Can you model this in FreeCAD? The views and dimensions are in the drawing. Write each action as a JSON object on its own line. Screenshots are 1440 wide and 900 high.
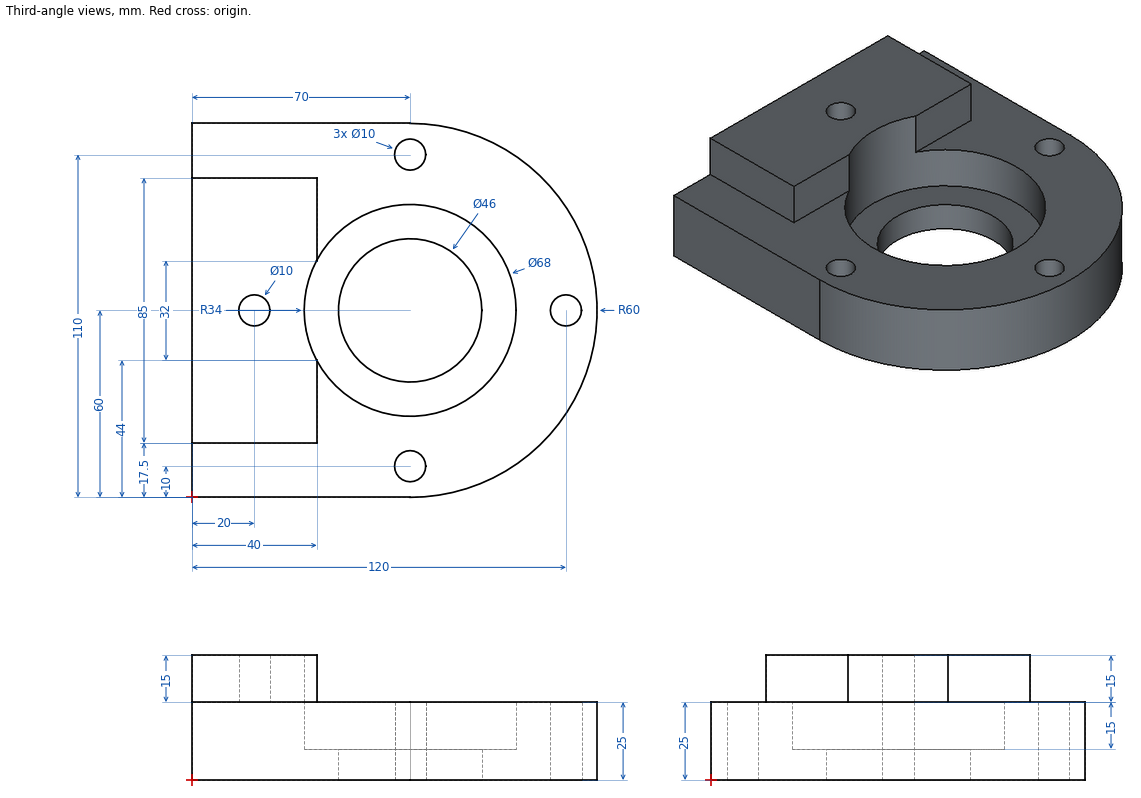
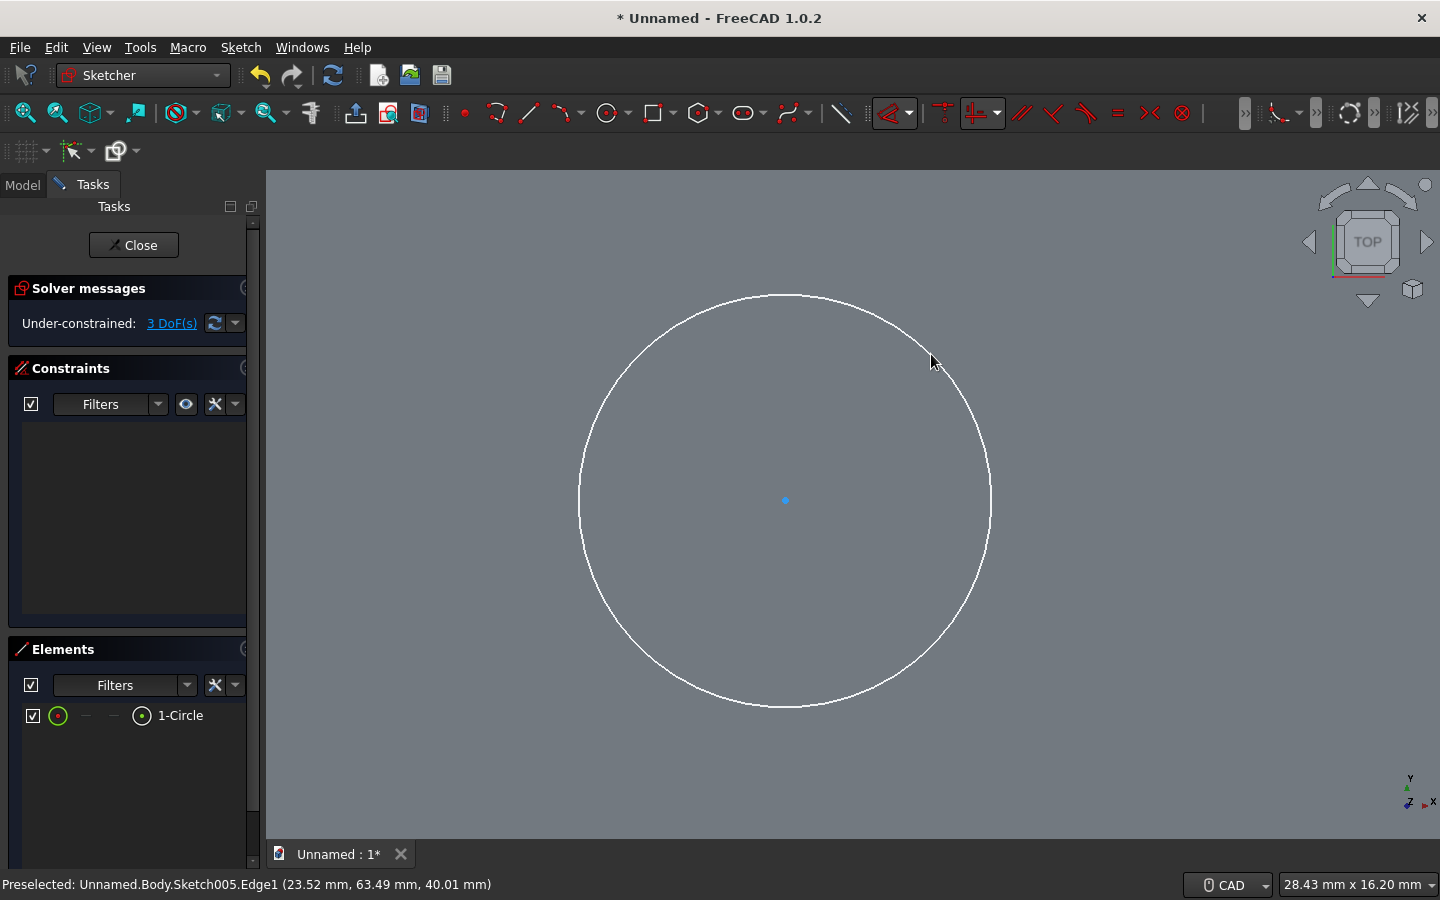
{"action": "left_click", "coordinate": [931, 355]}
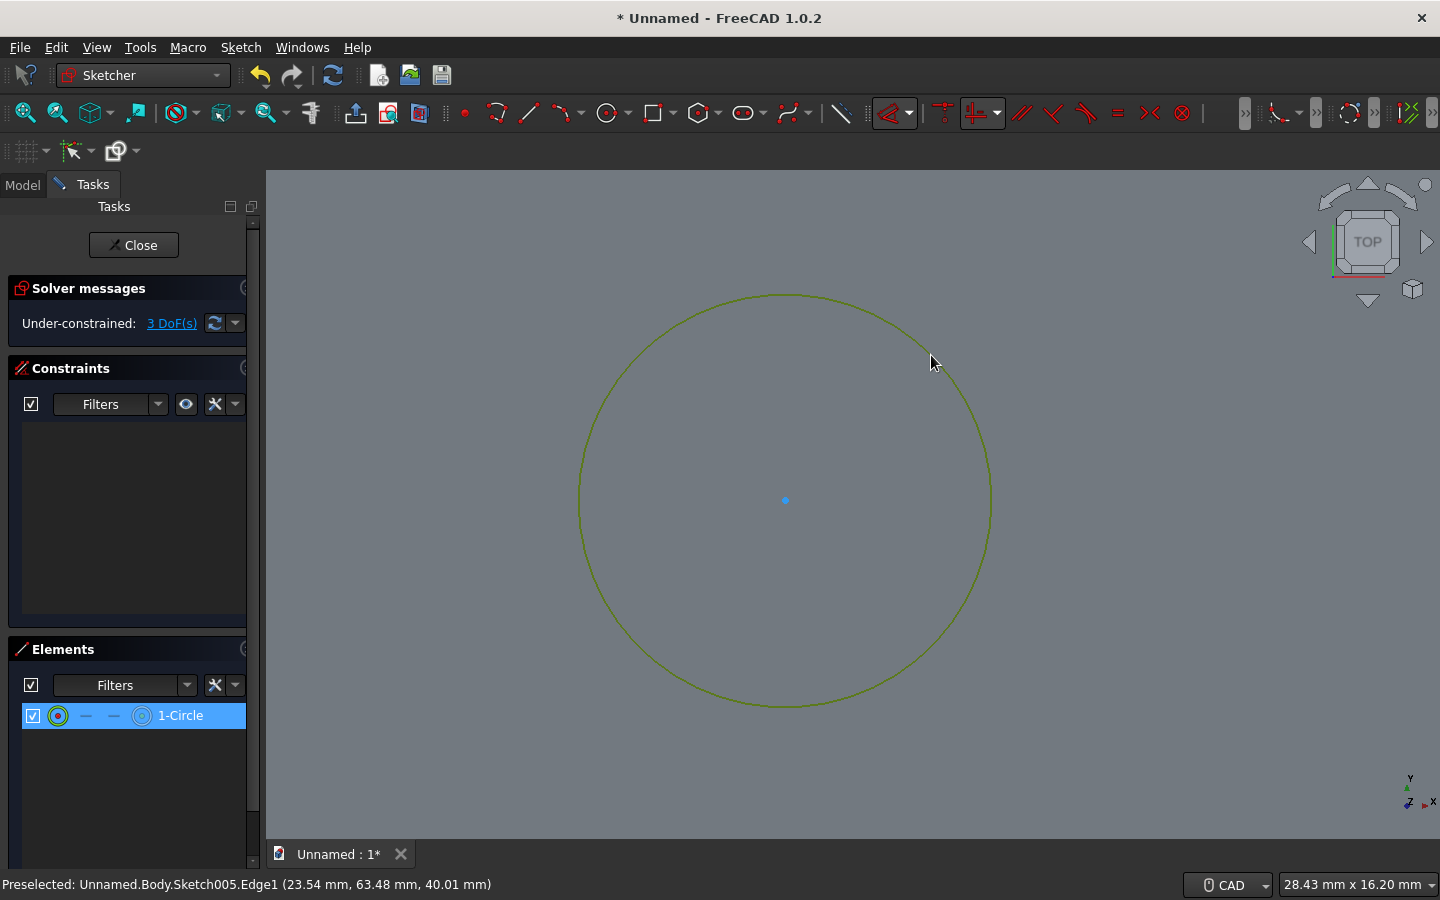
{"action": "key", "text": "k o"}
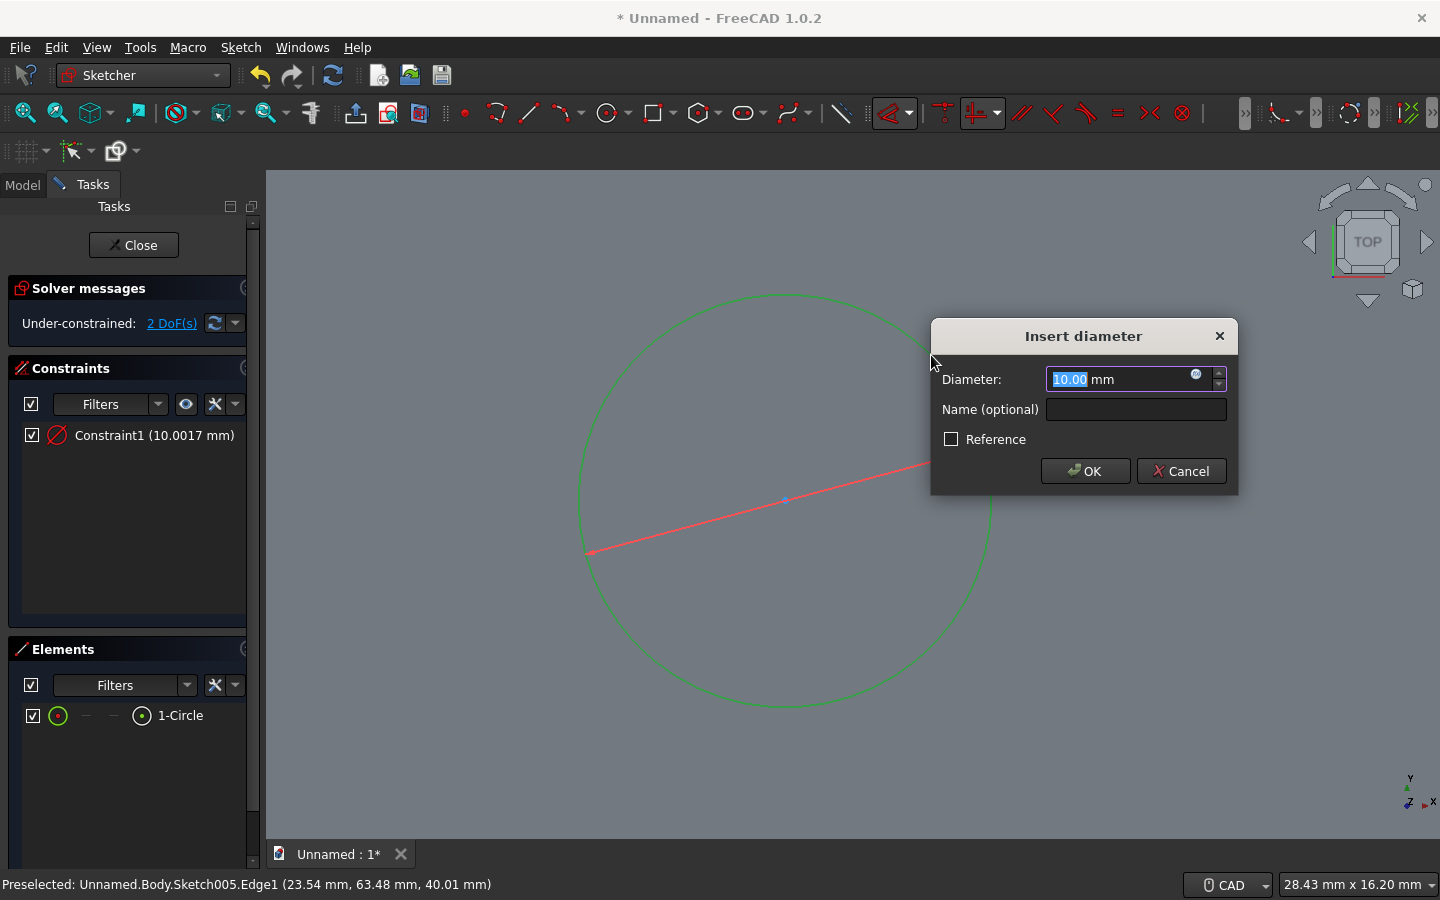
{"action": "type", "text": "10"}
{"action": "key", "text": "Return"}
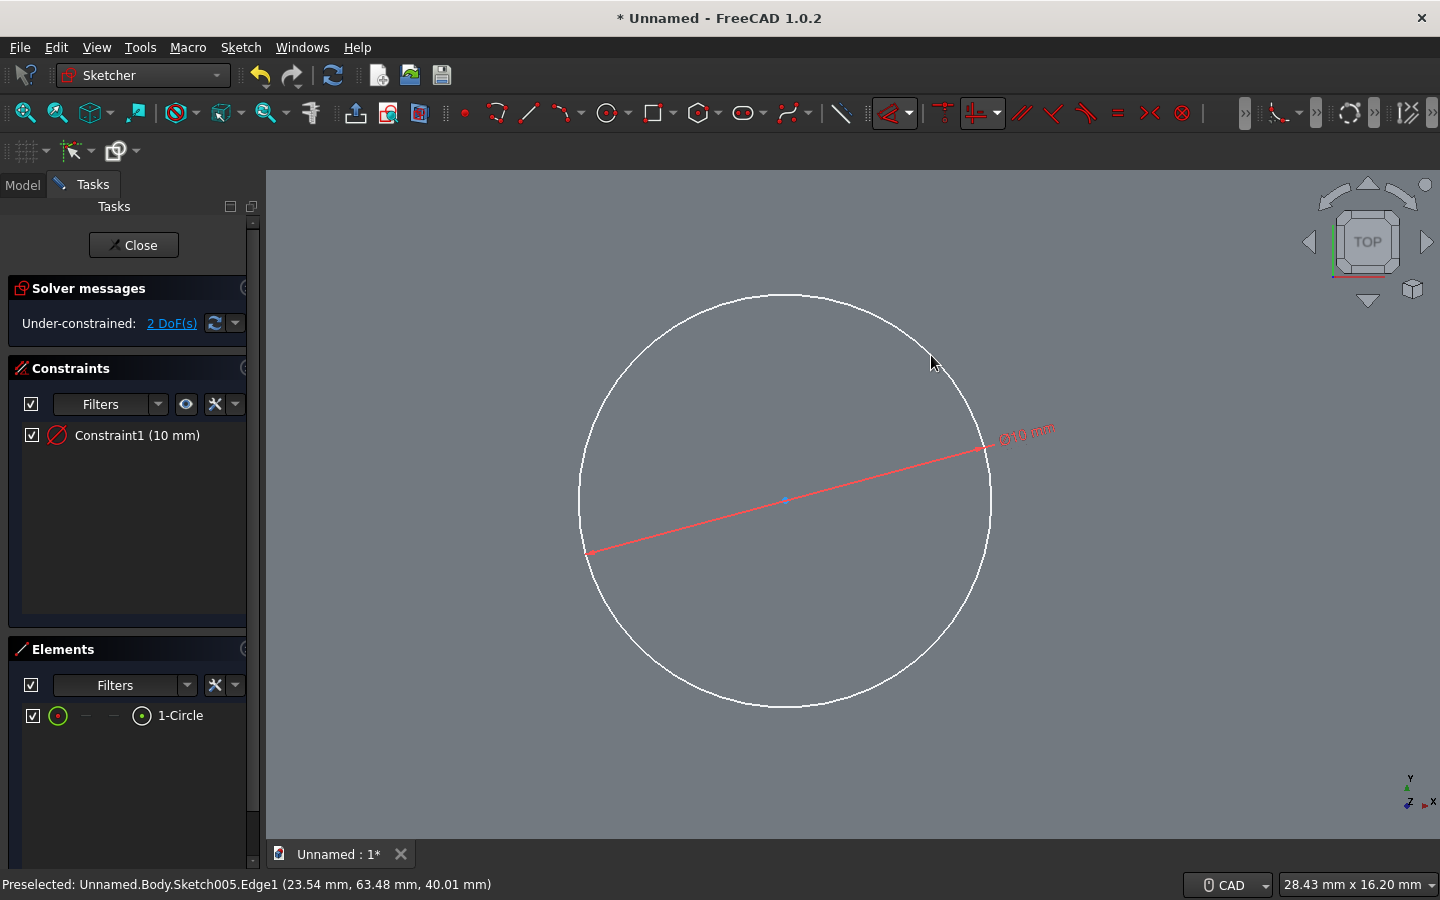
{"action": "left_click", "coordinate": [785, 501]}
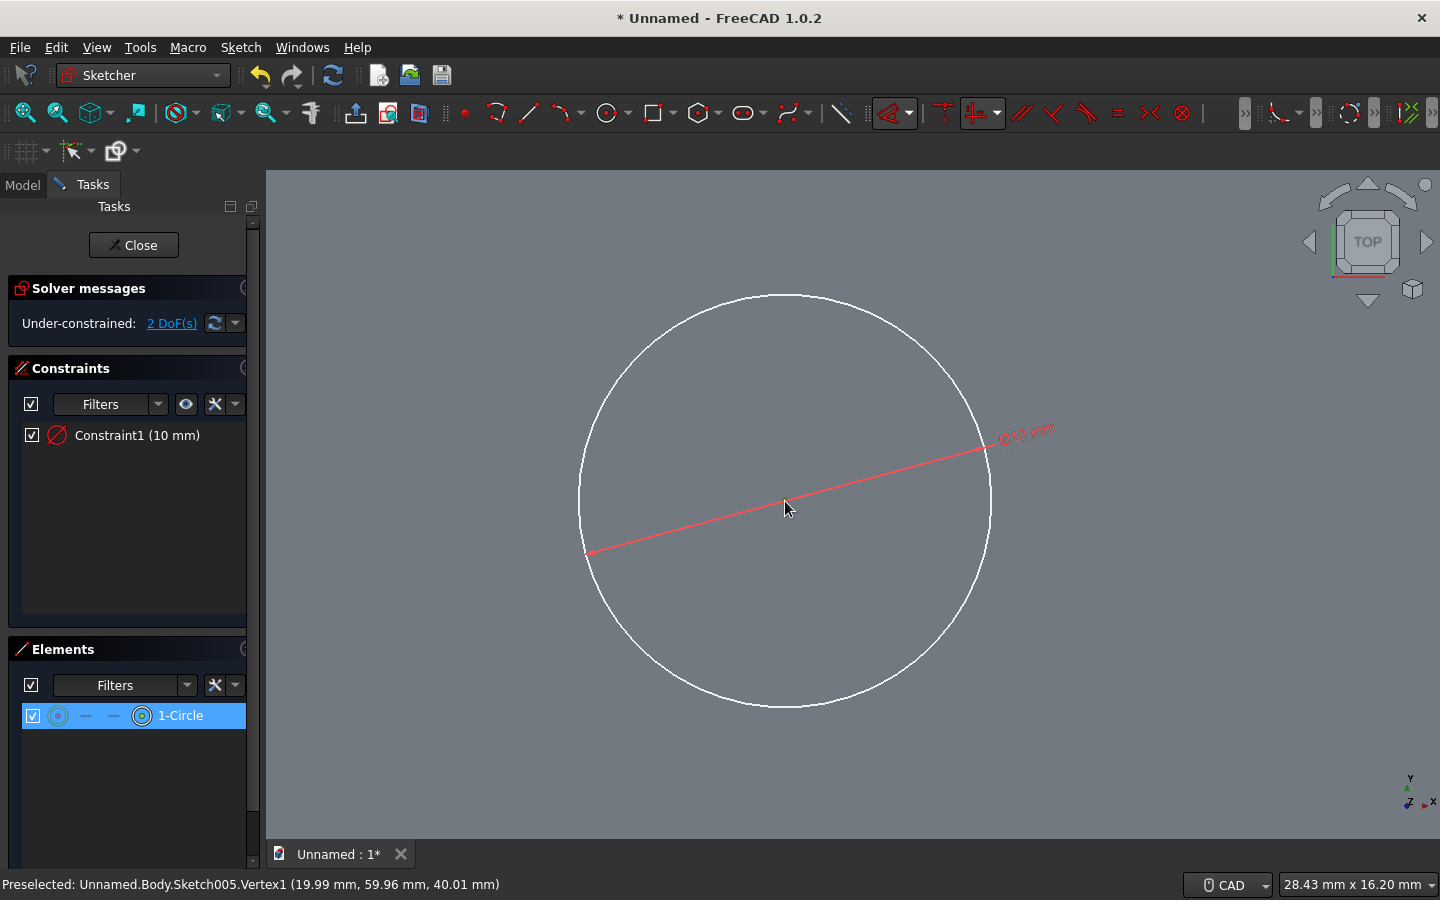
{"action": "left_click", "coordinate": [912, 114]}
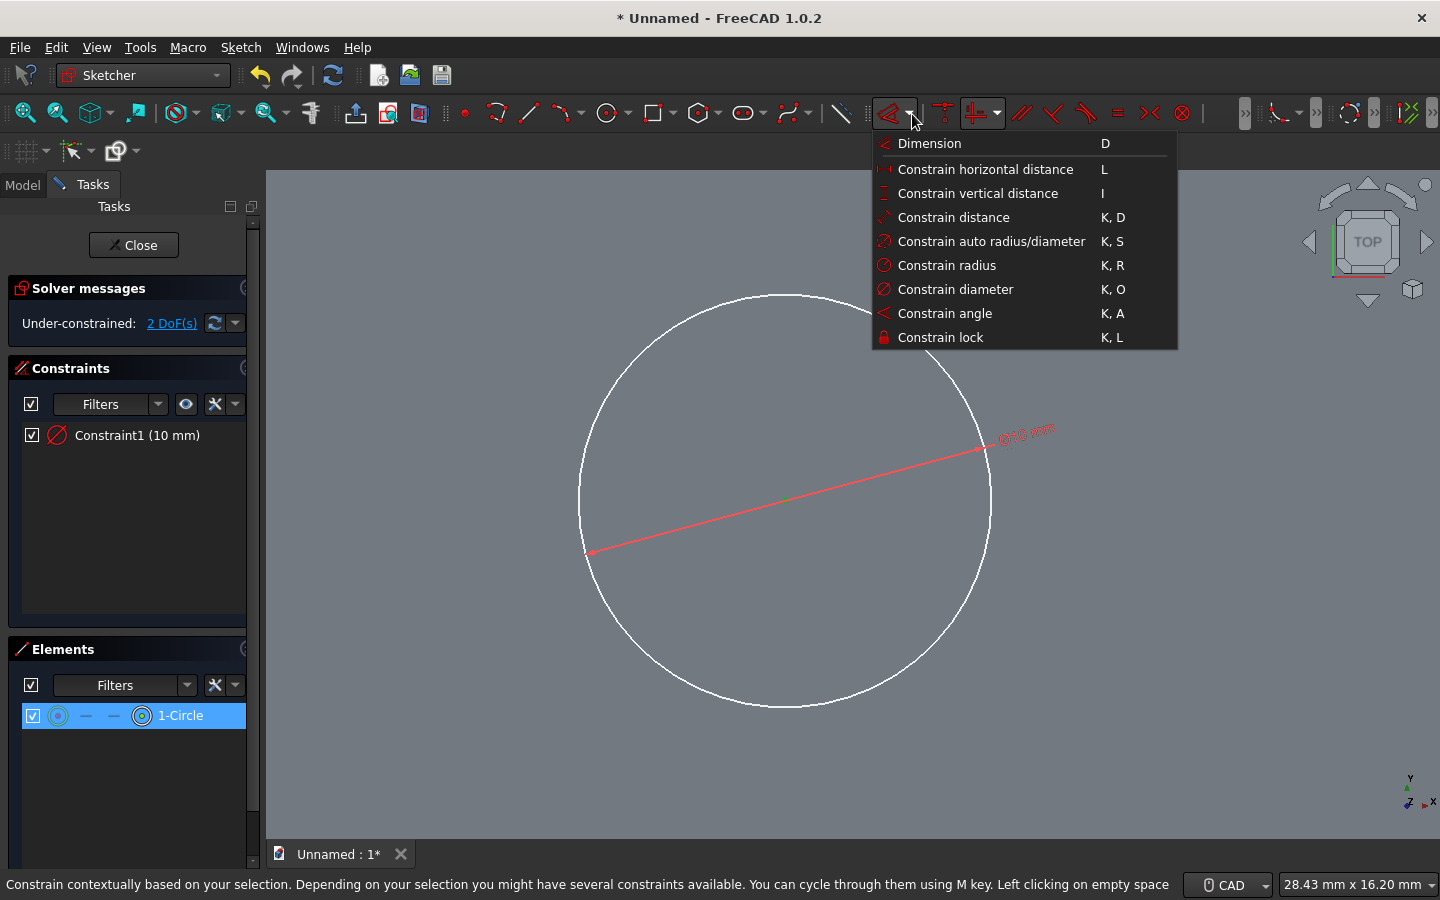
{"action": "left_click", "coordinate": [1025, 169]}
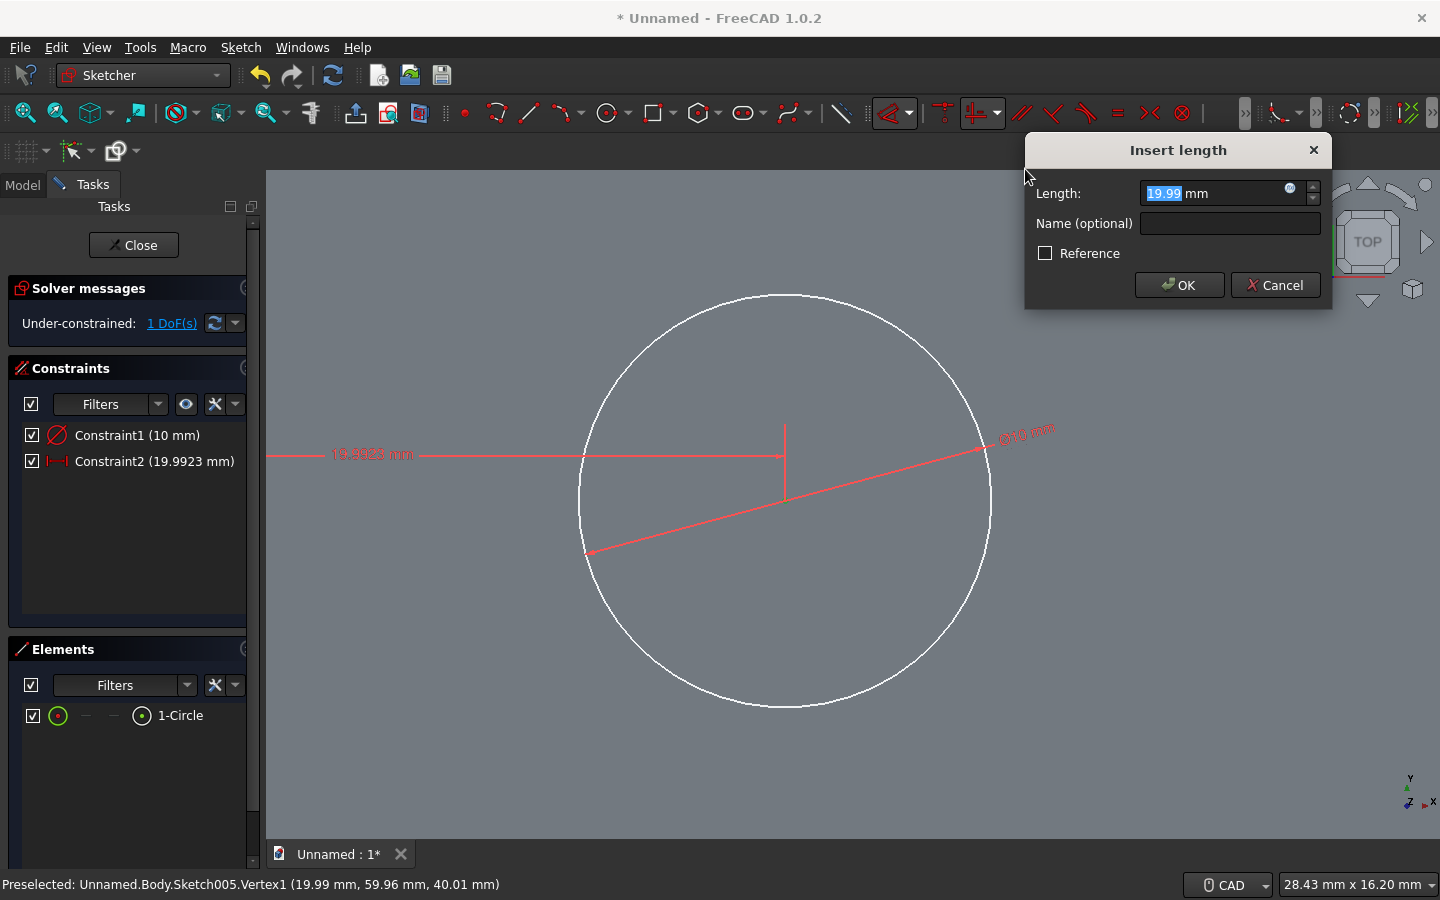
{"action": "type", "text": "20"}
{"action": "key", "text": "Return"}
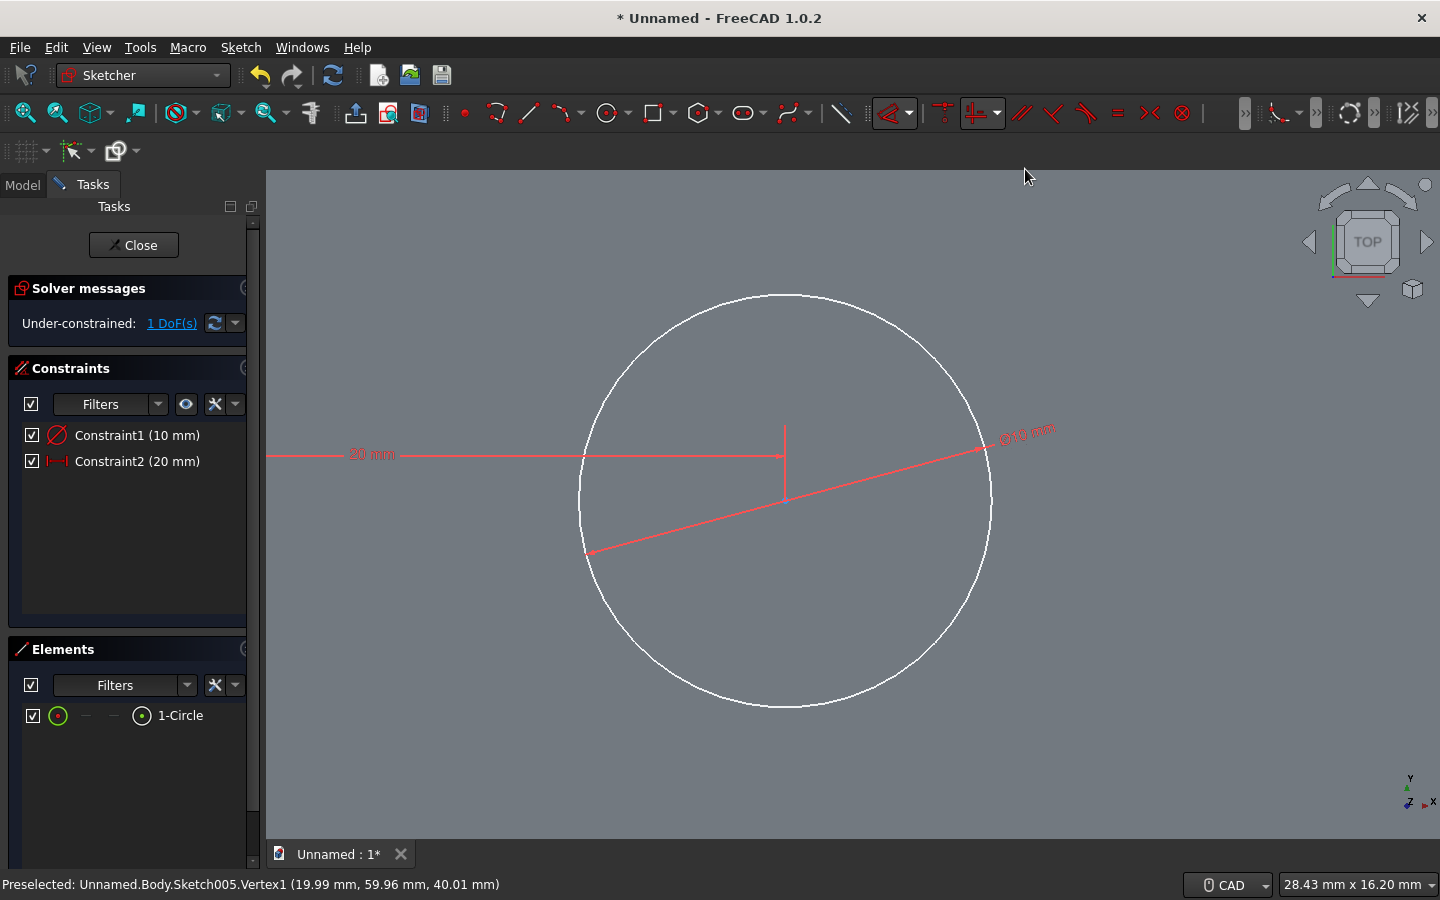
{"action": "left_click", "coordinate": [785, 501]}